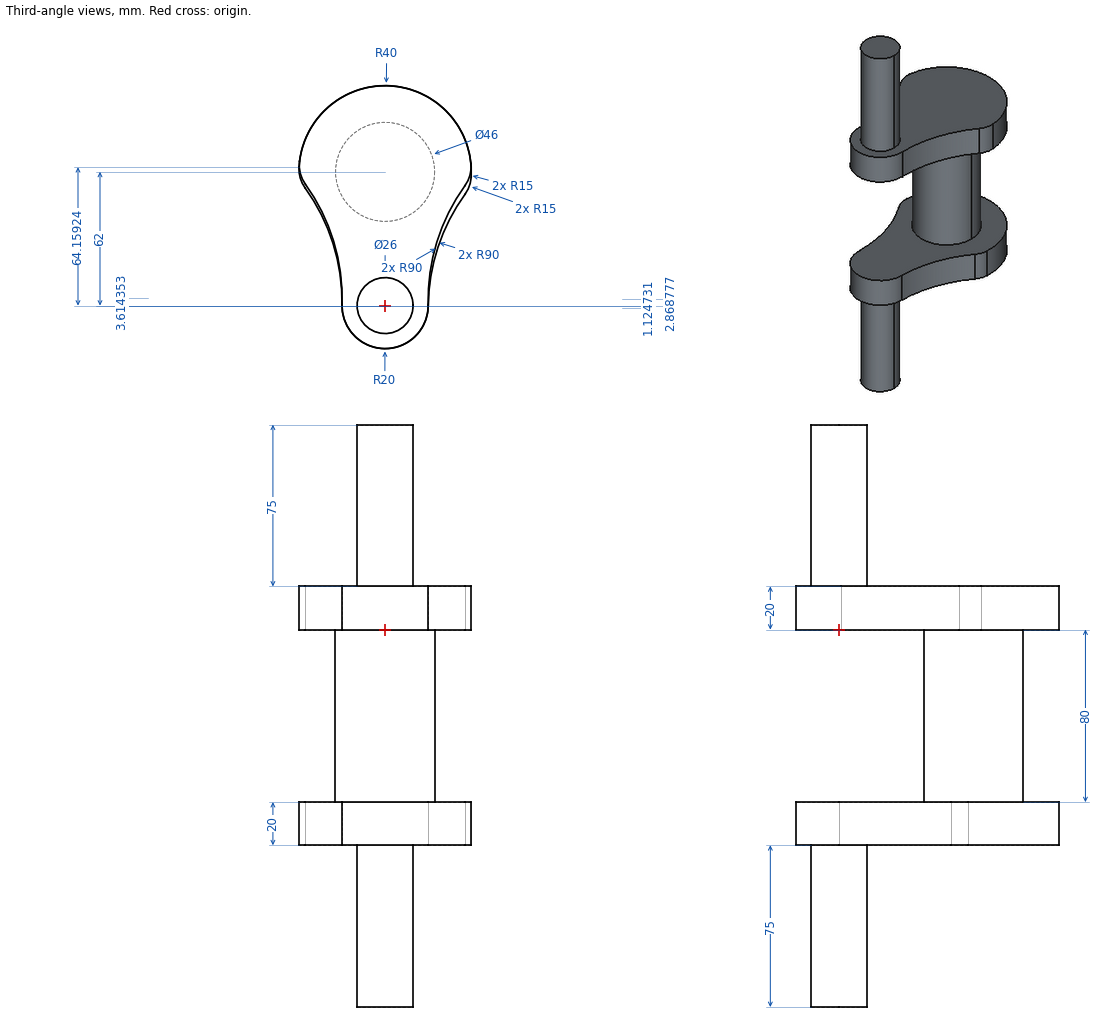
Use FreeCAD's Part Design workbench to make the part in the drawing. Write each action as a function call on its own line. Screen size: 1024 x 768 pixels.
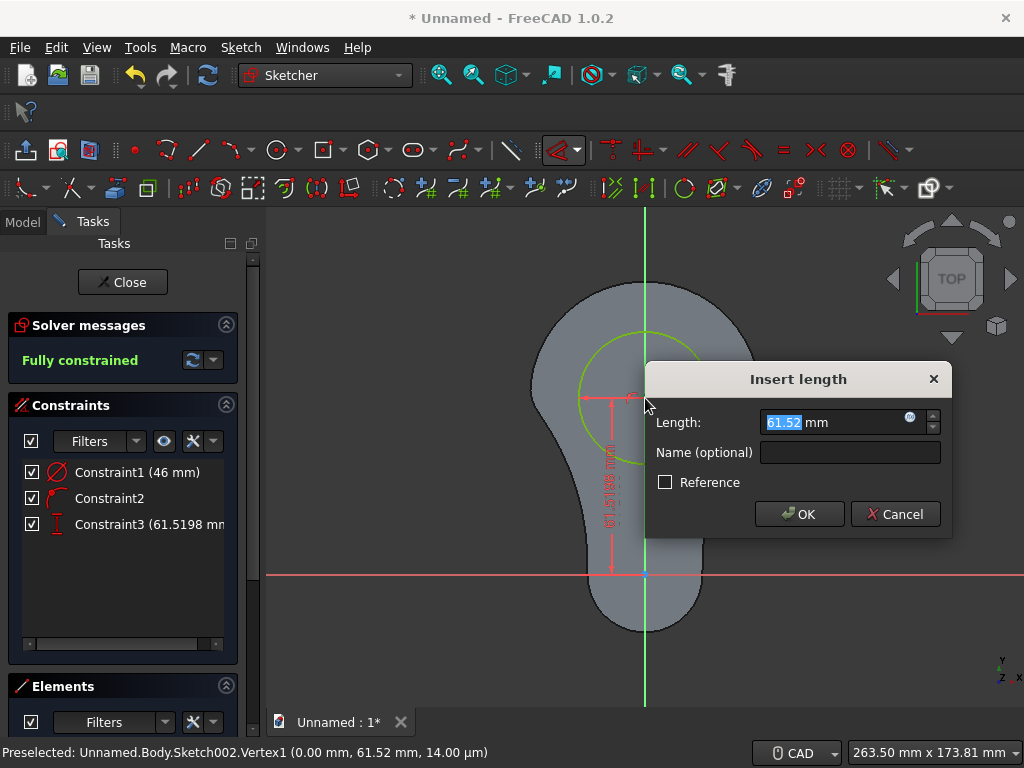
text(62)
key(Return)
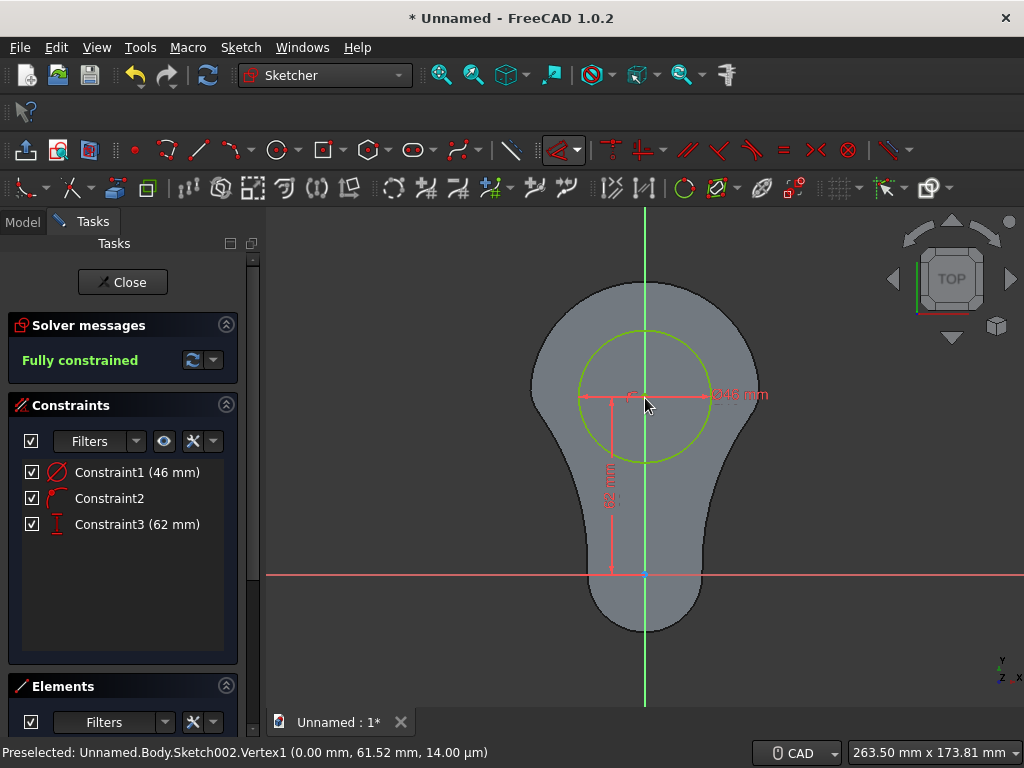
click(123, 282)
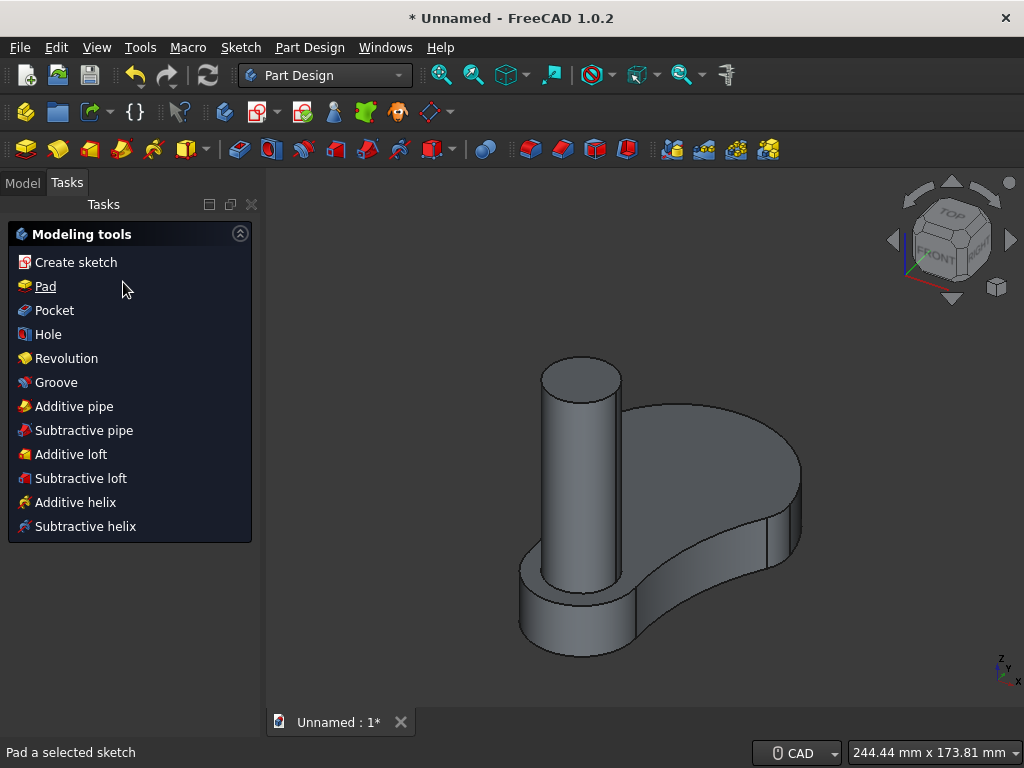
click(26, 150)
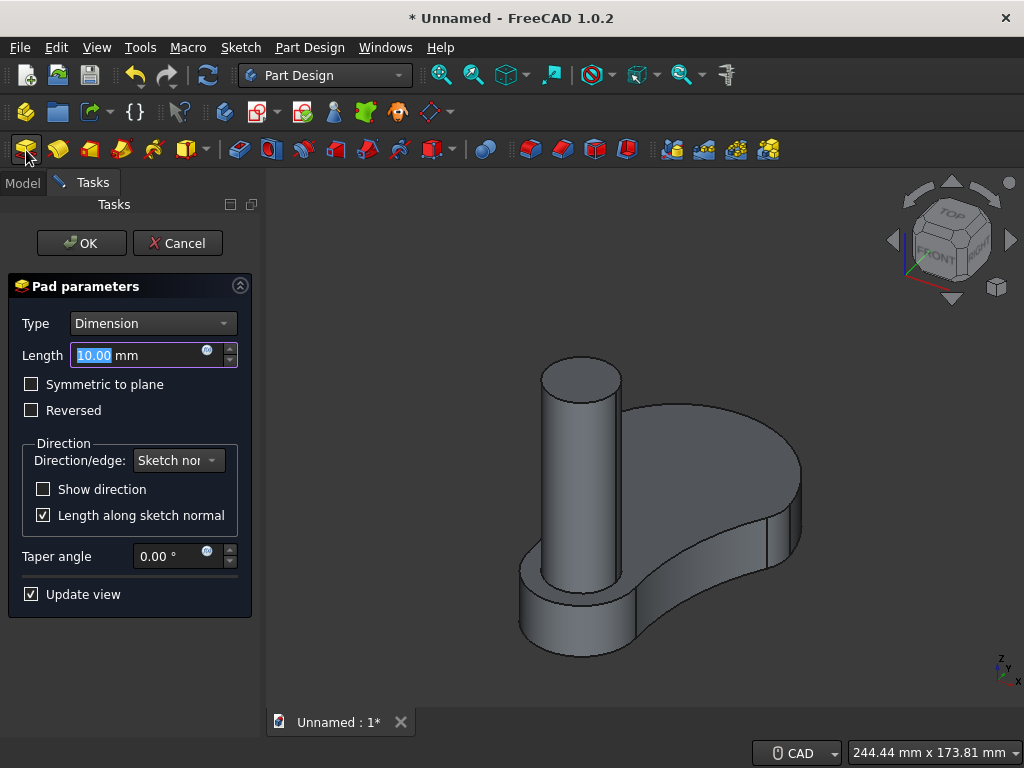
text(80)
key(Tab)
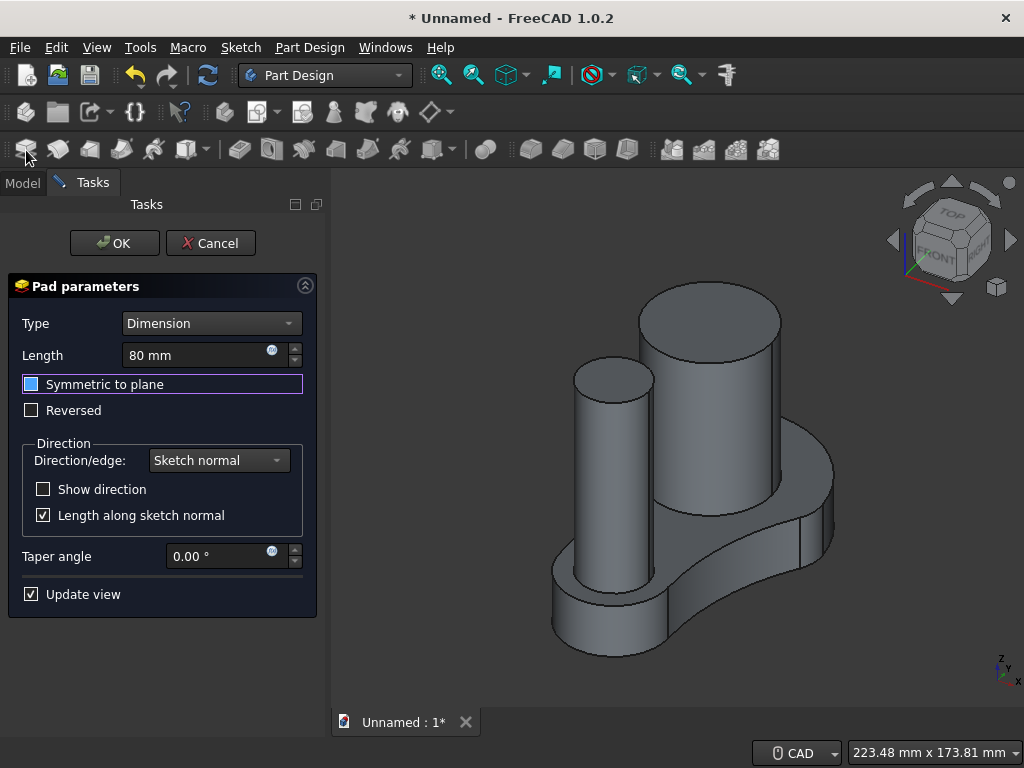
click(30, 410)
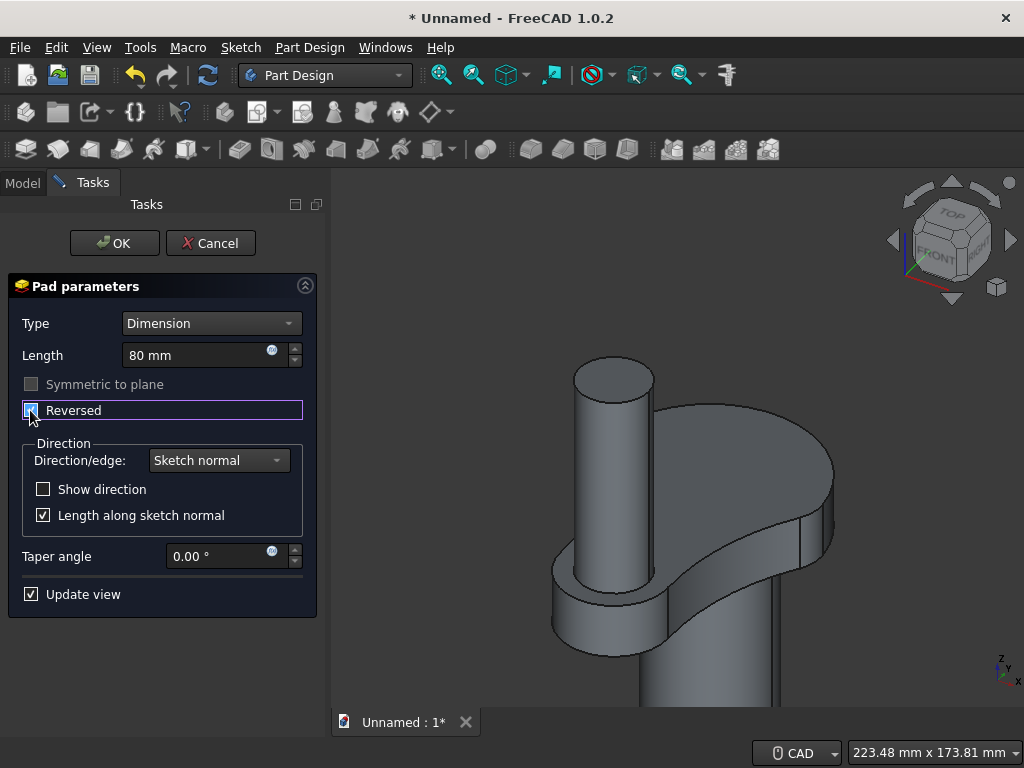
click(115, 243)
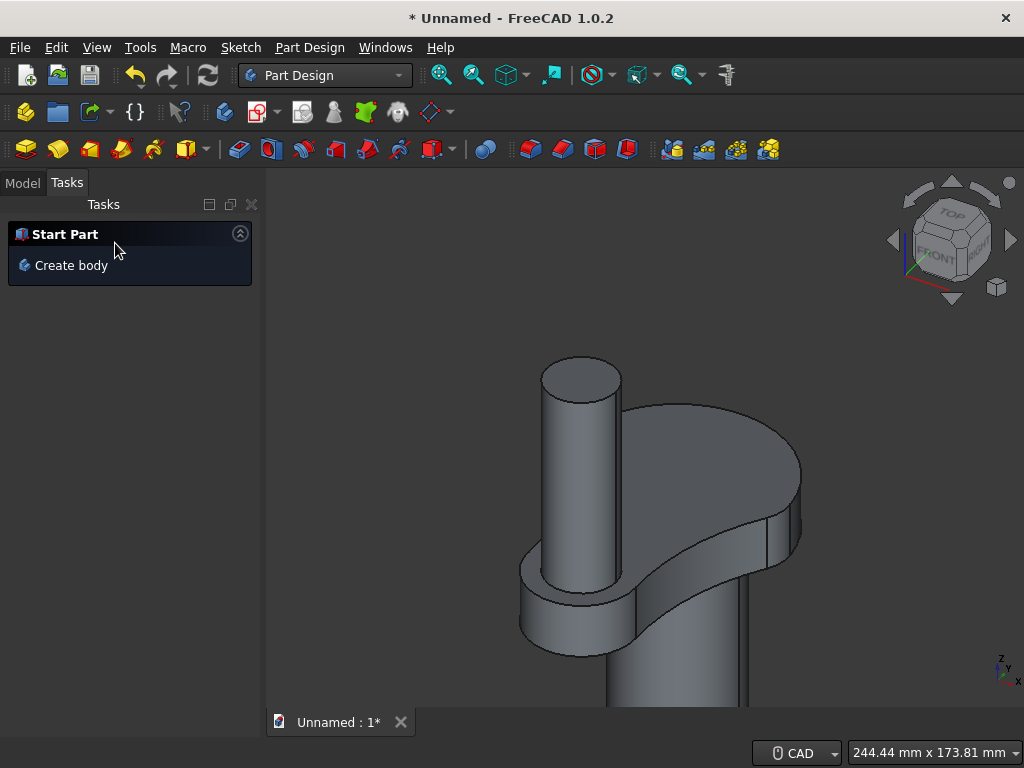
click(442, 76)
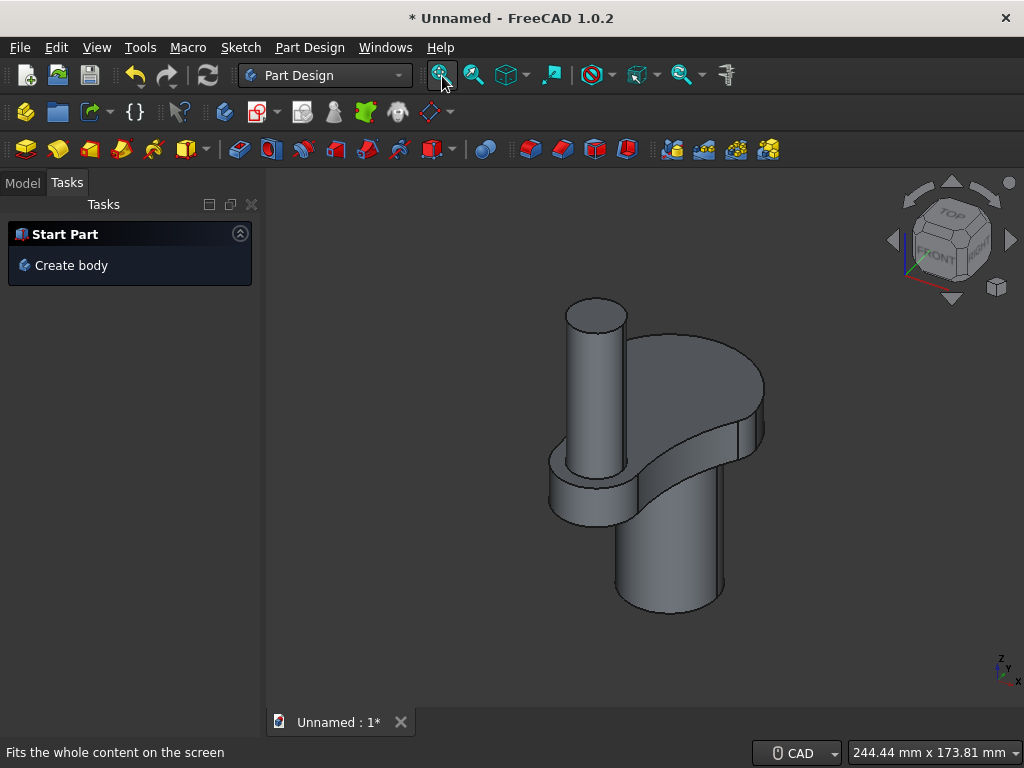
click(23, 182)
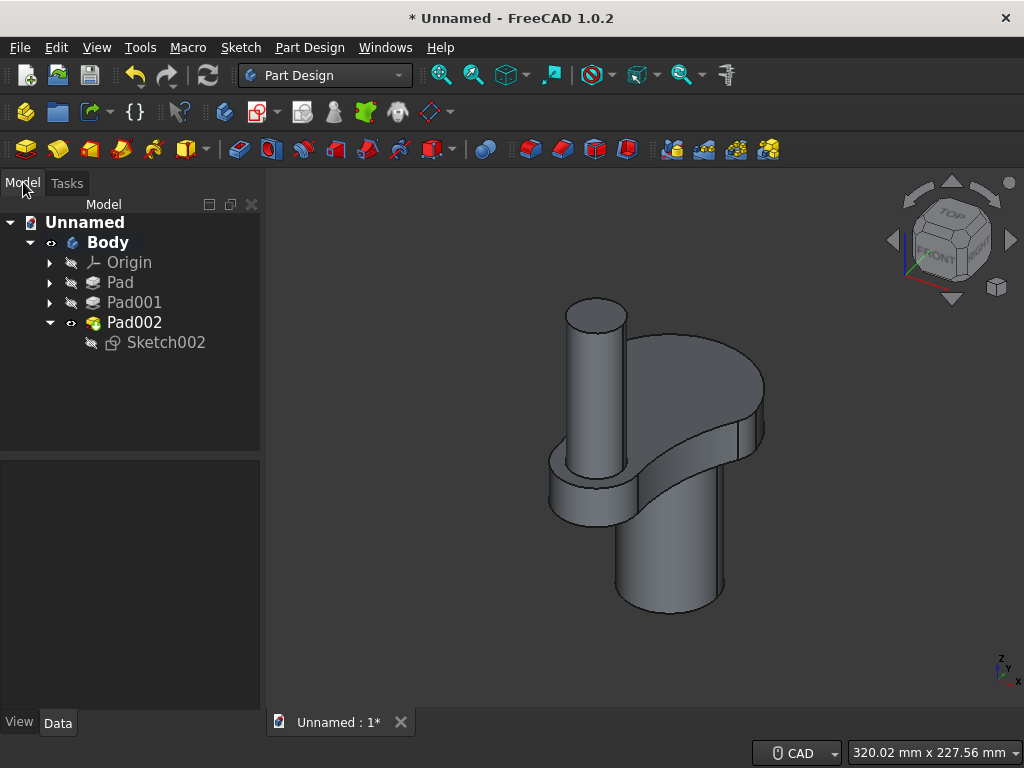
click(50, 263)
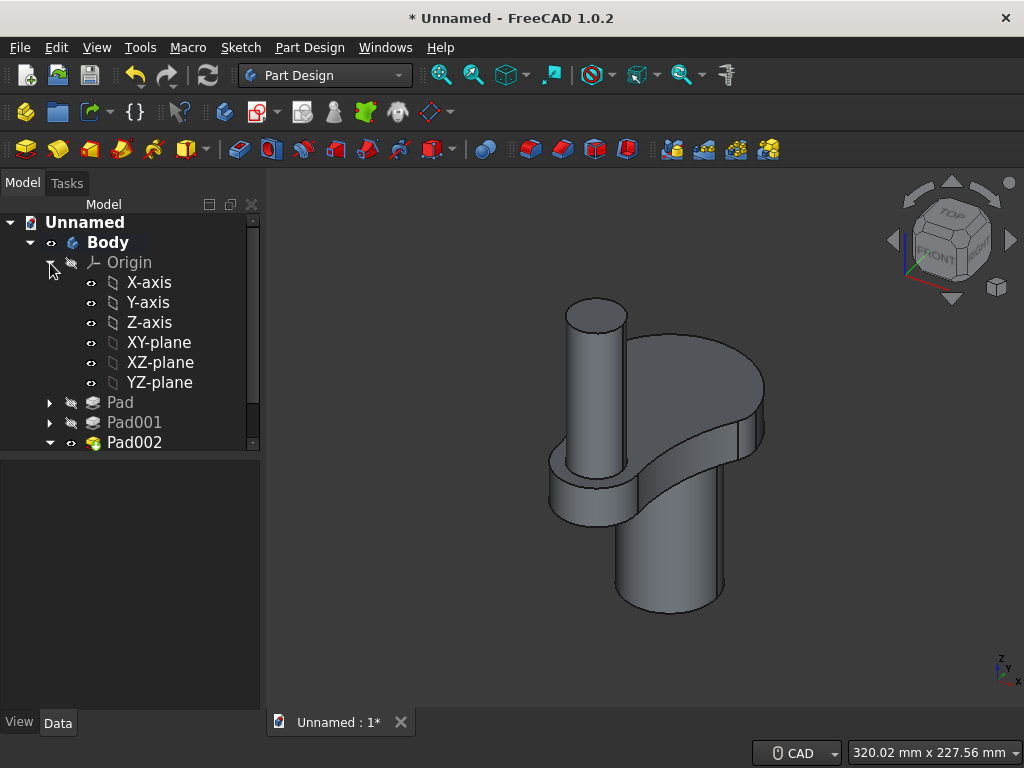
click(136, 343)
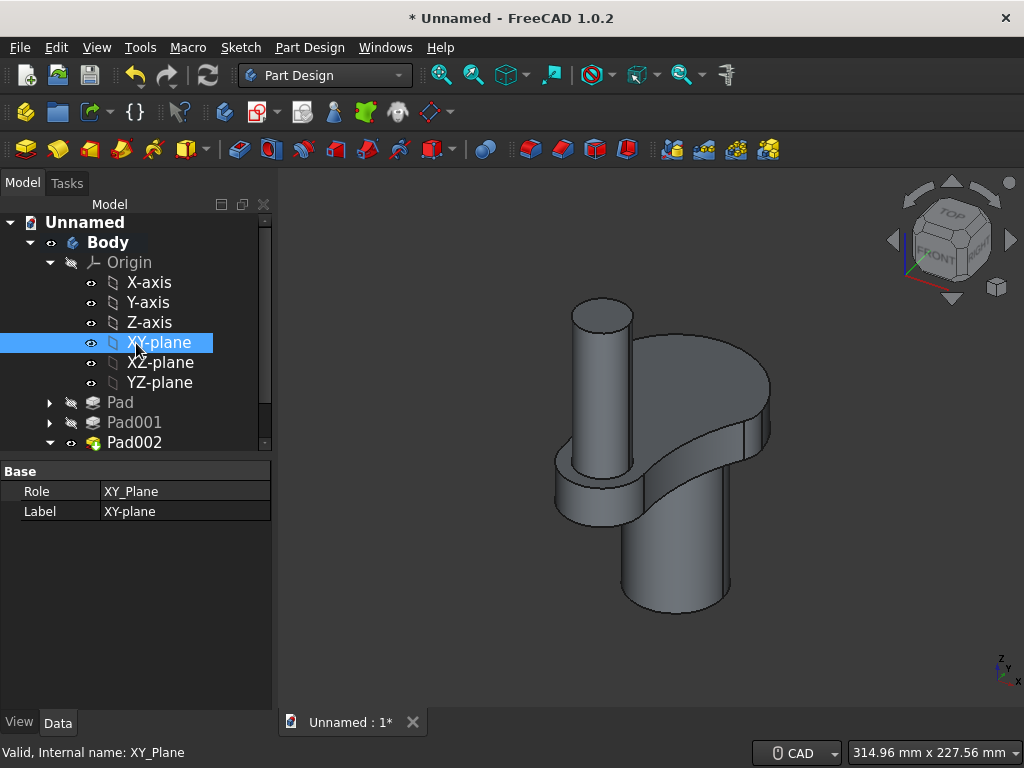
click(430, 112)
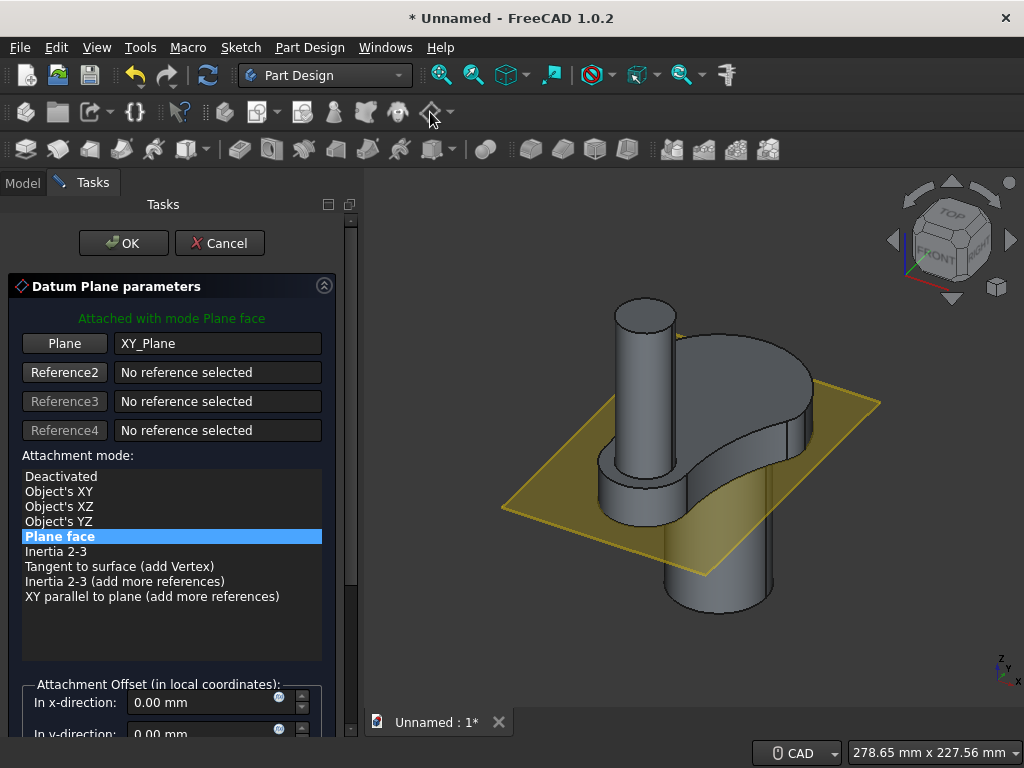
scroll(351, 475, down, 2)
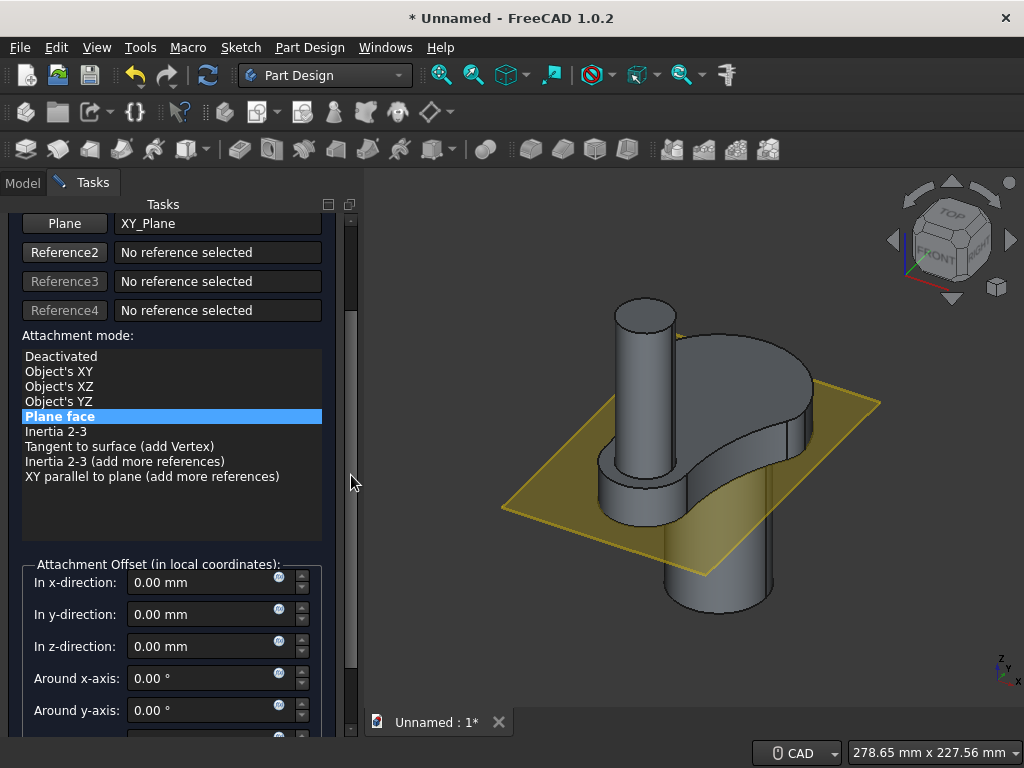
triple_click(210, 646)